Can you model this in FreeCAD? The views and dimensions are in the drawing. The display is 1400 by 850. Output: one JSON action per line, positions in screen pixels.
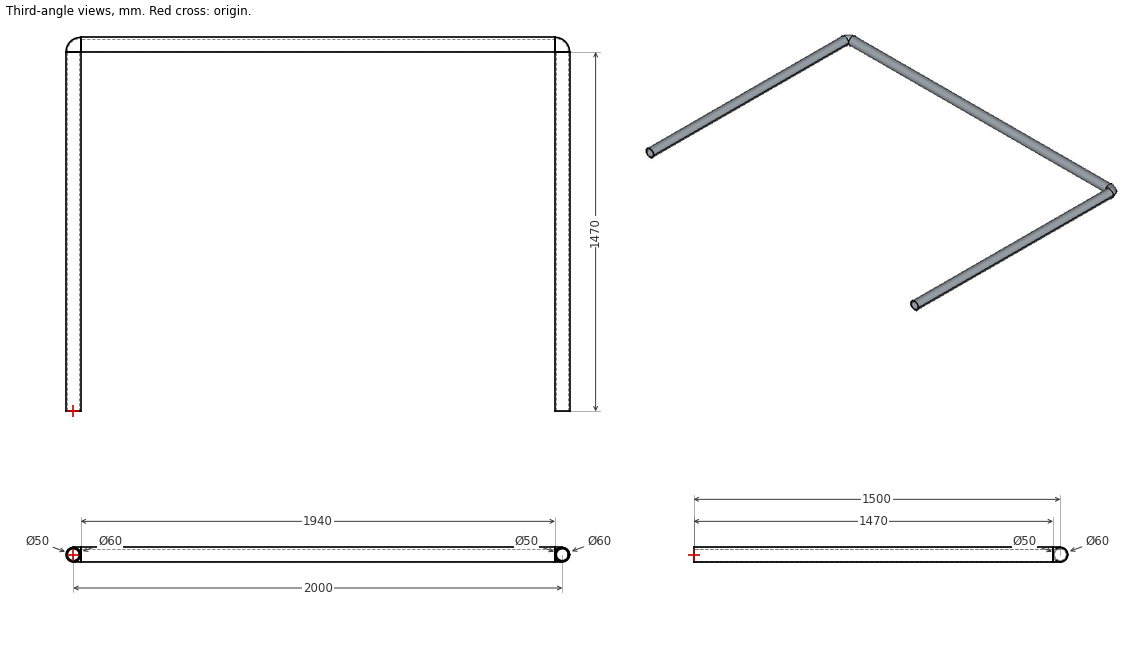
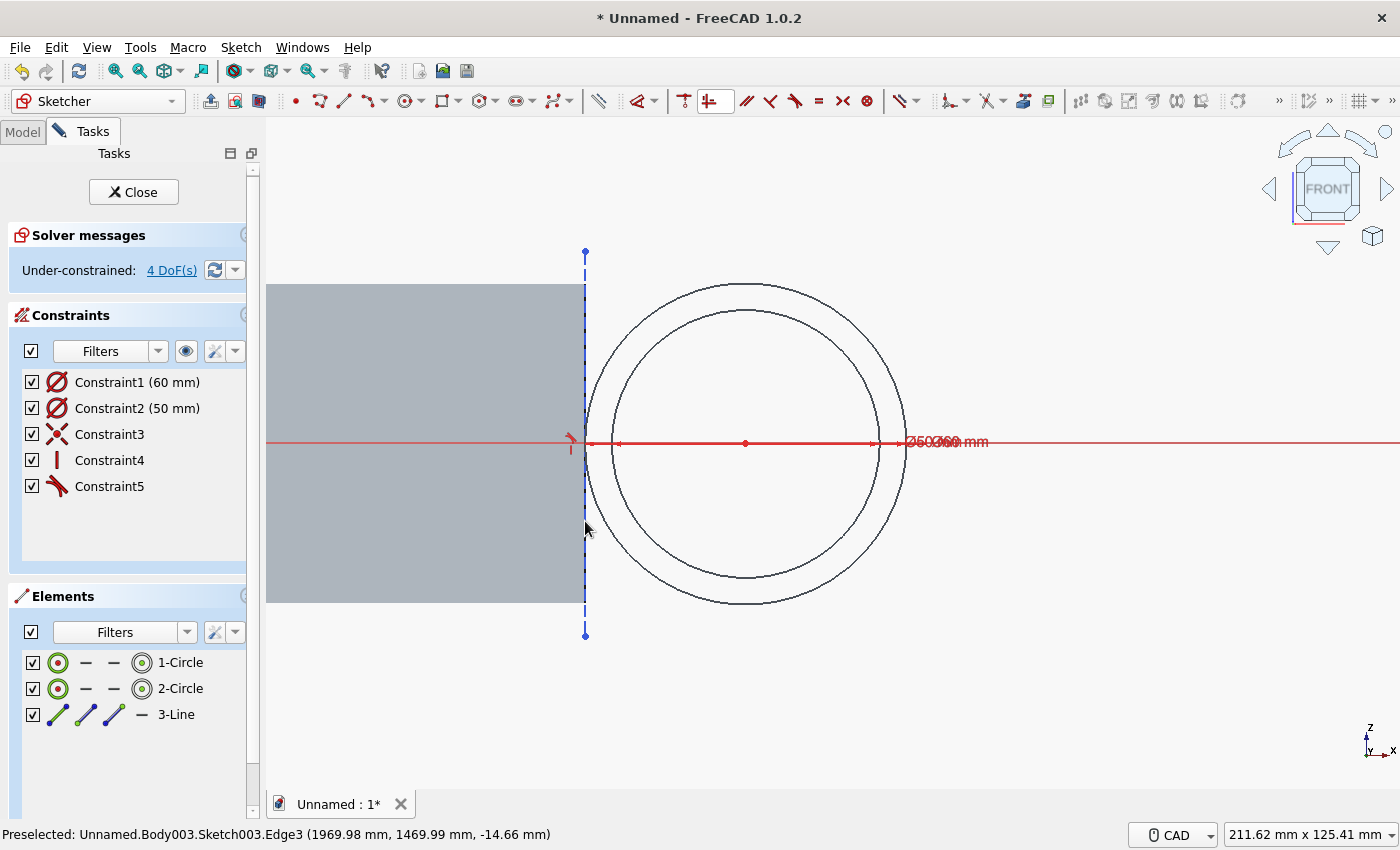
{"action": "left_click", "coordinate": [746, 444]}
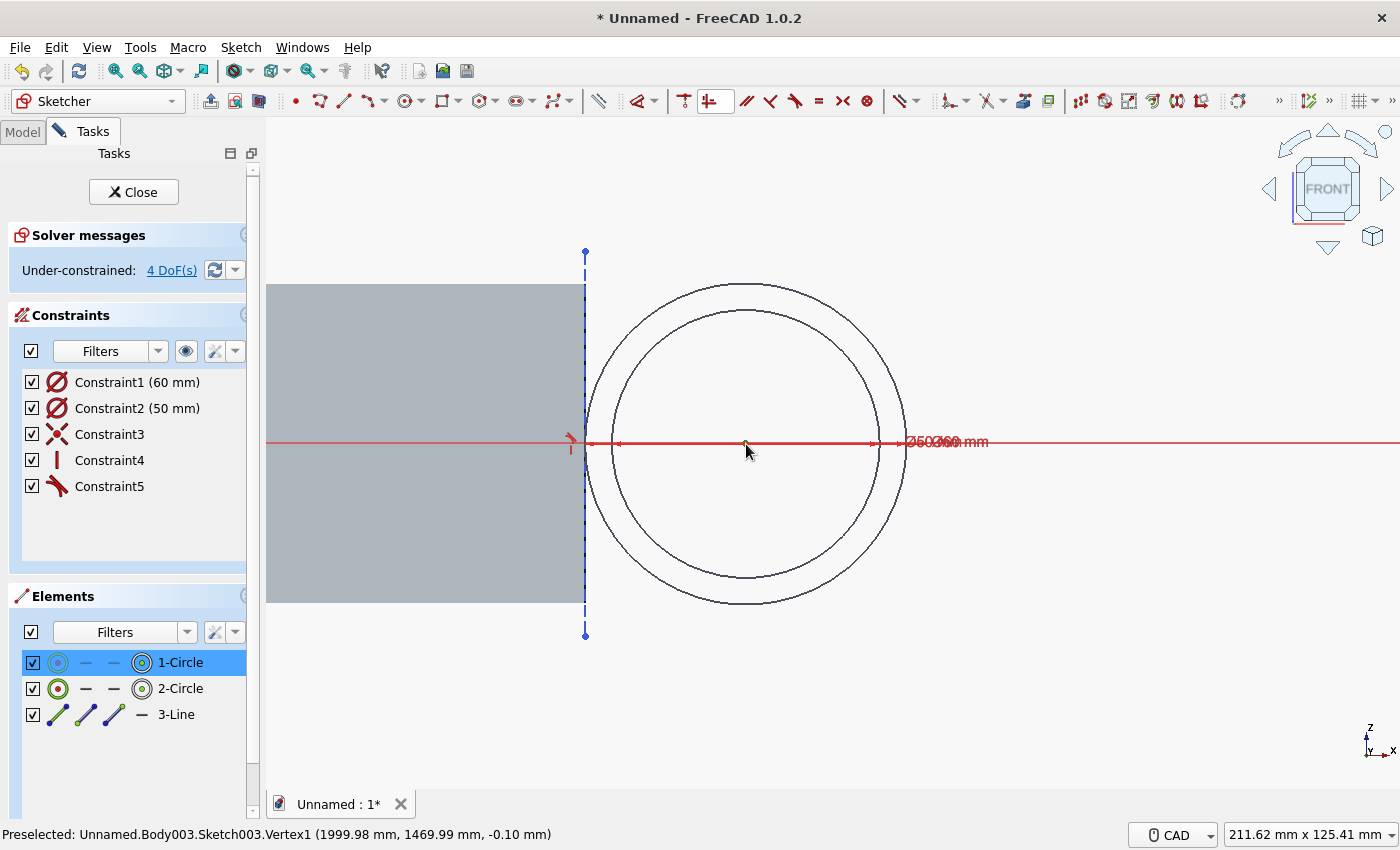
{"action": "left_click", "coordinate": [361, 443]}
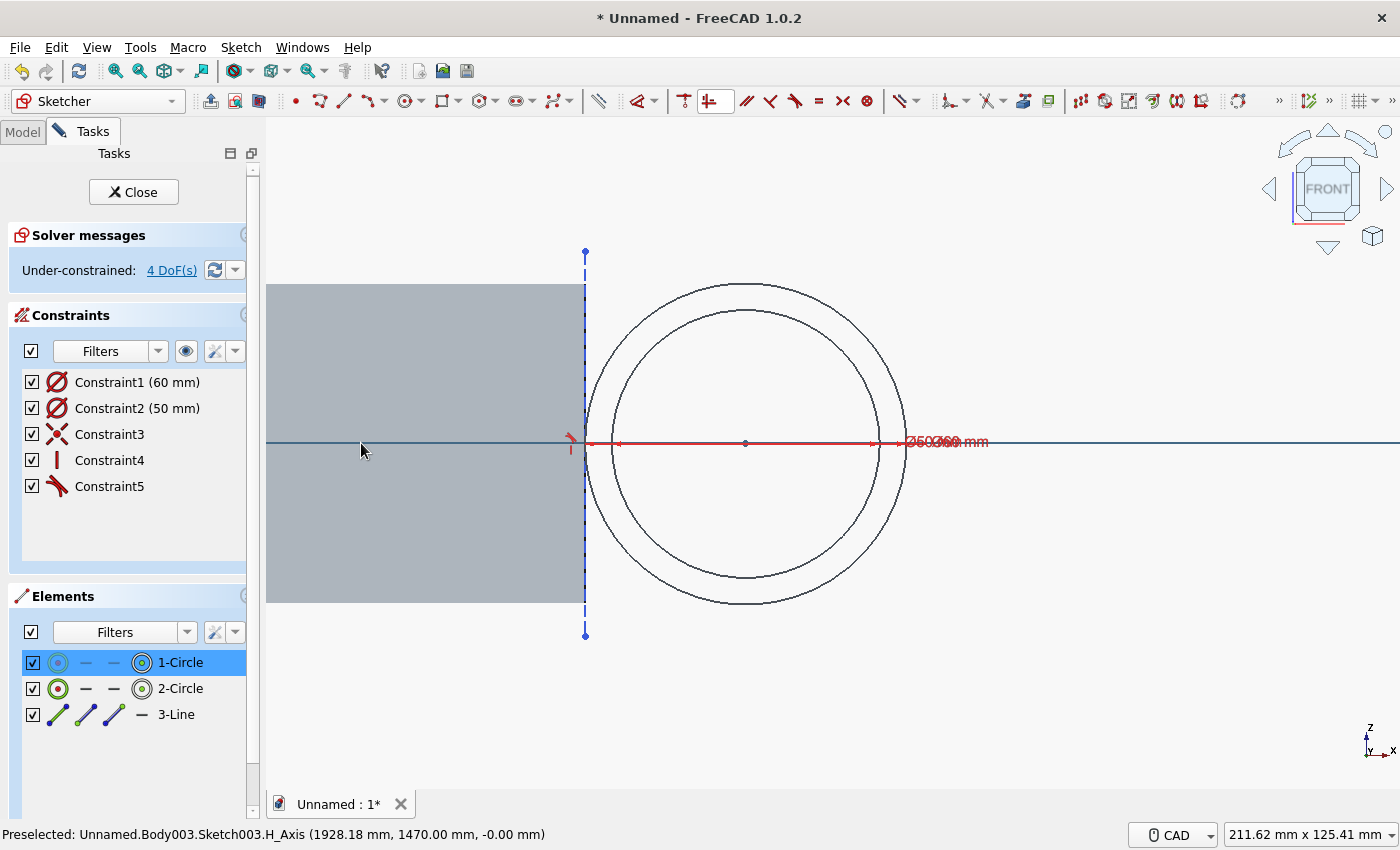
{"action": "key", "text": "c"}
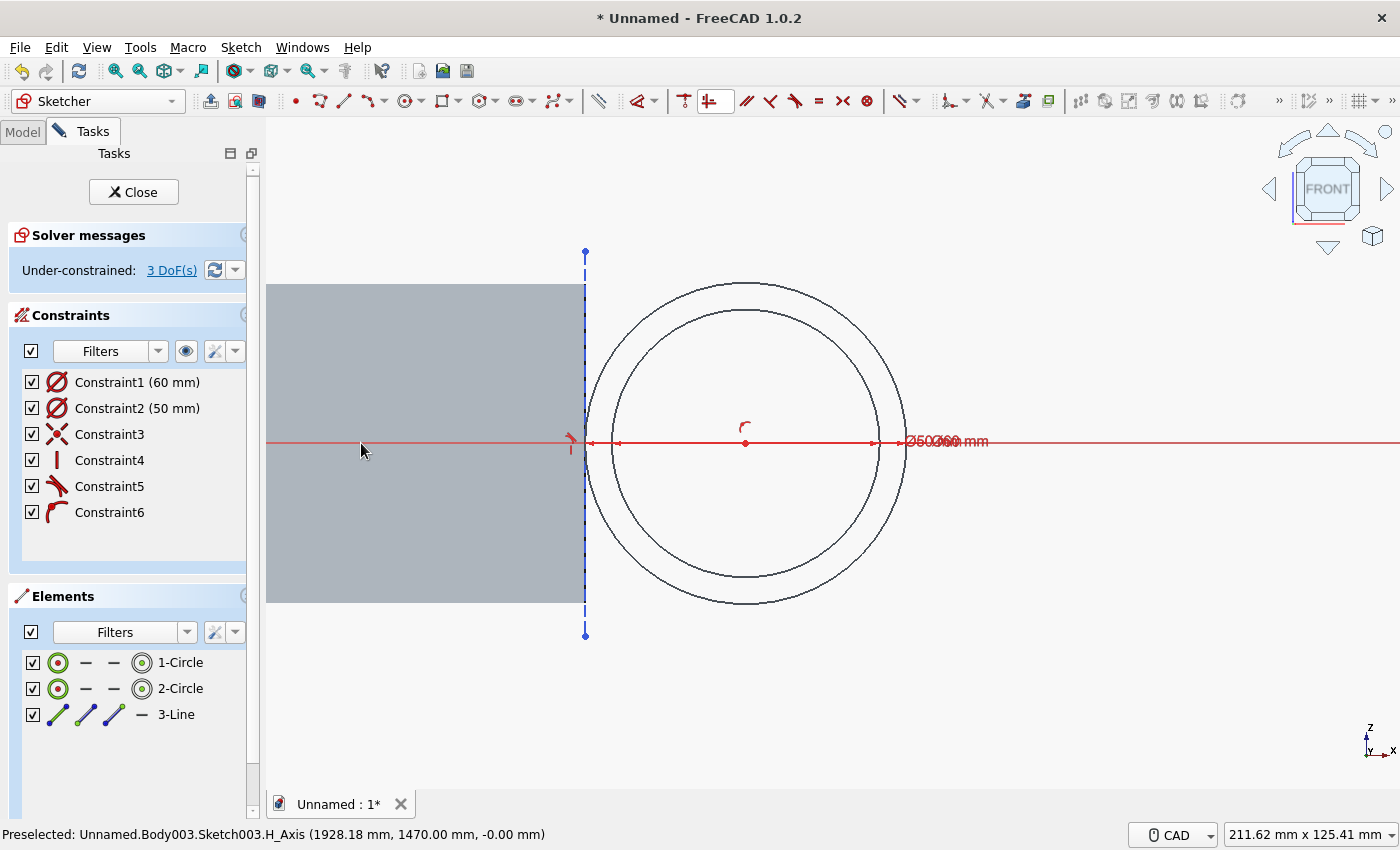
{"action": "left_click", "coordinate": [638, 102]}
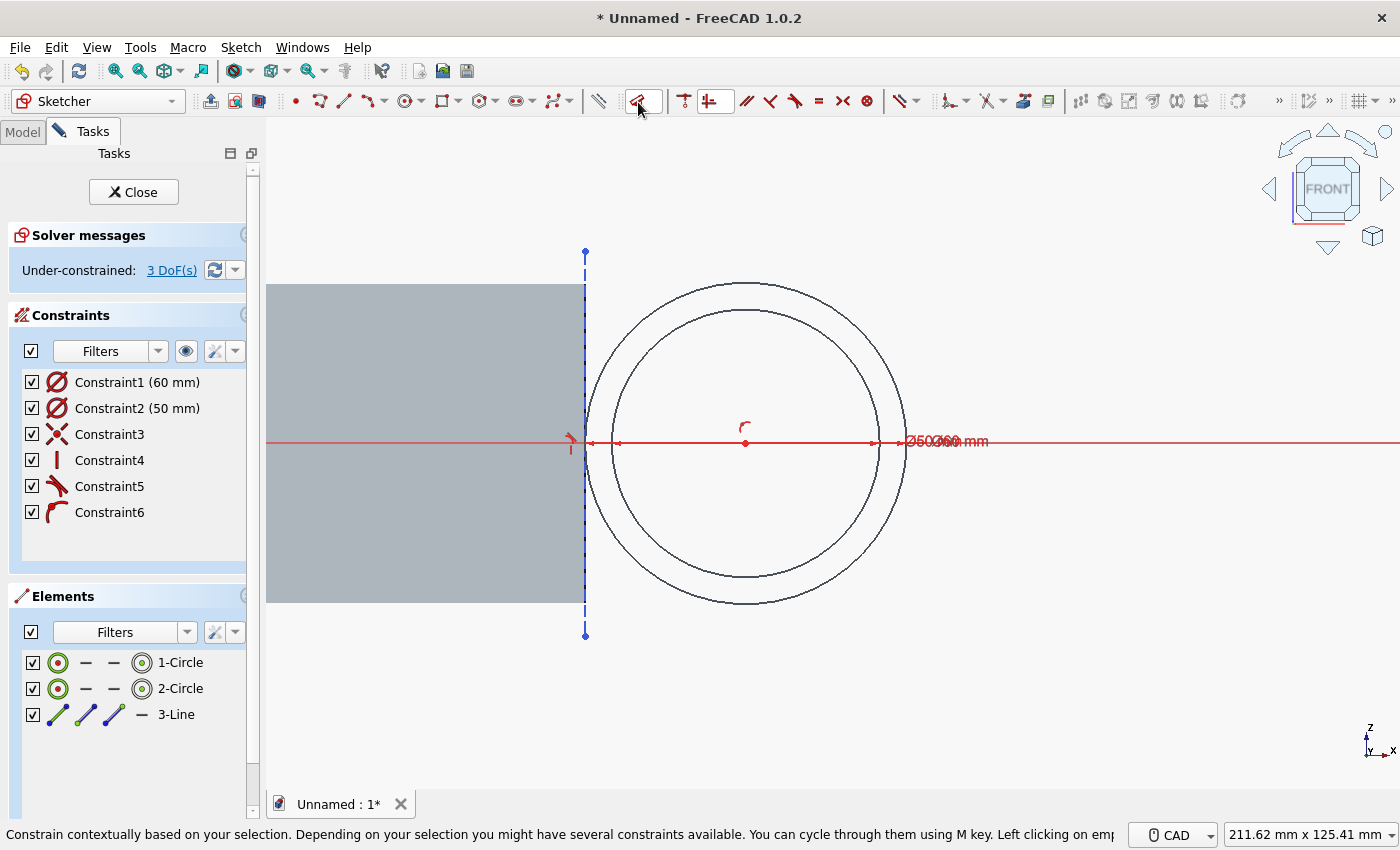
{"action": "left_click", "coordinate": [746, 443]}
{"action": "left_click", "coordinate": [520, 477]}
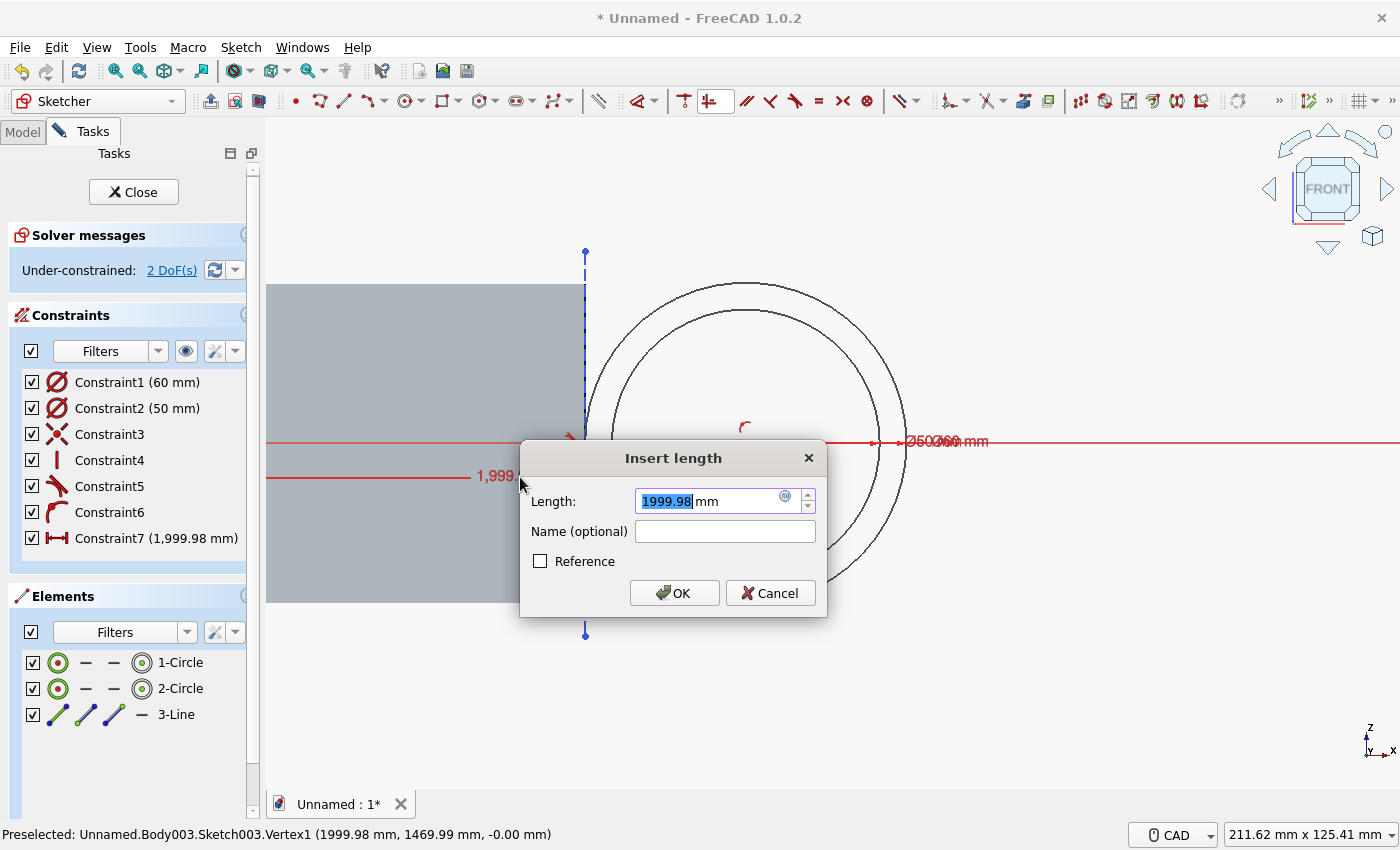
{"action": "type", "text": "2000"}
{"action": "key", "text": "Return"}
{"action": "key", "text": "Escape"}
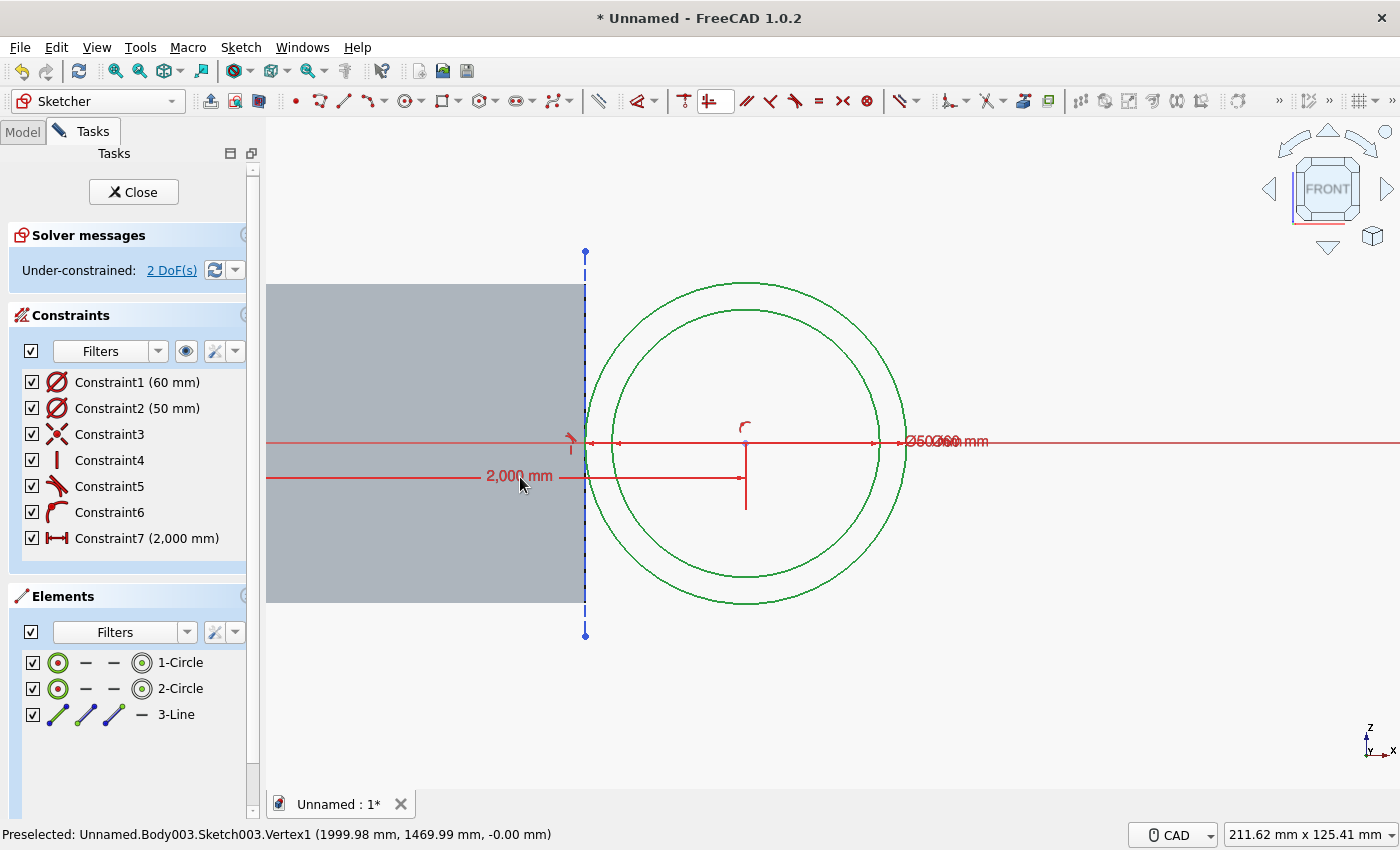
{"action": "left_click", "coordinate": [134, 192]}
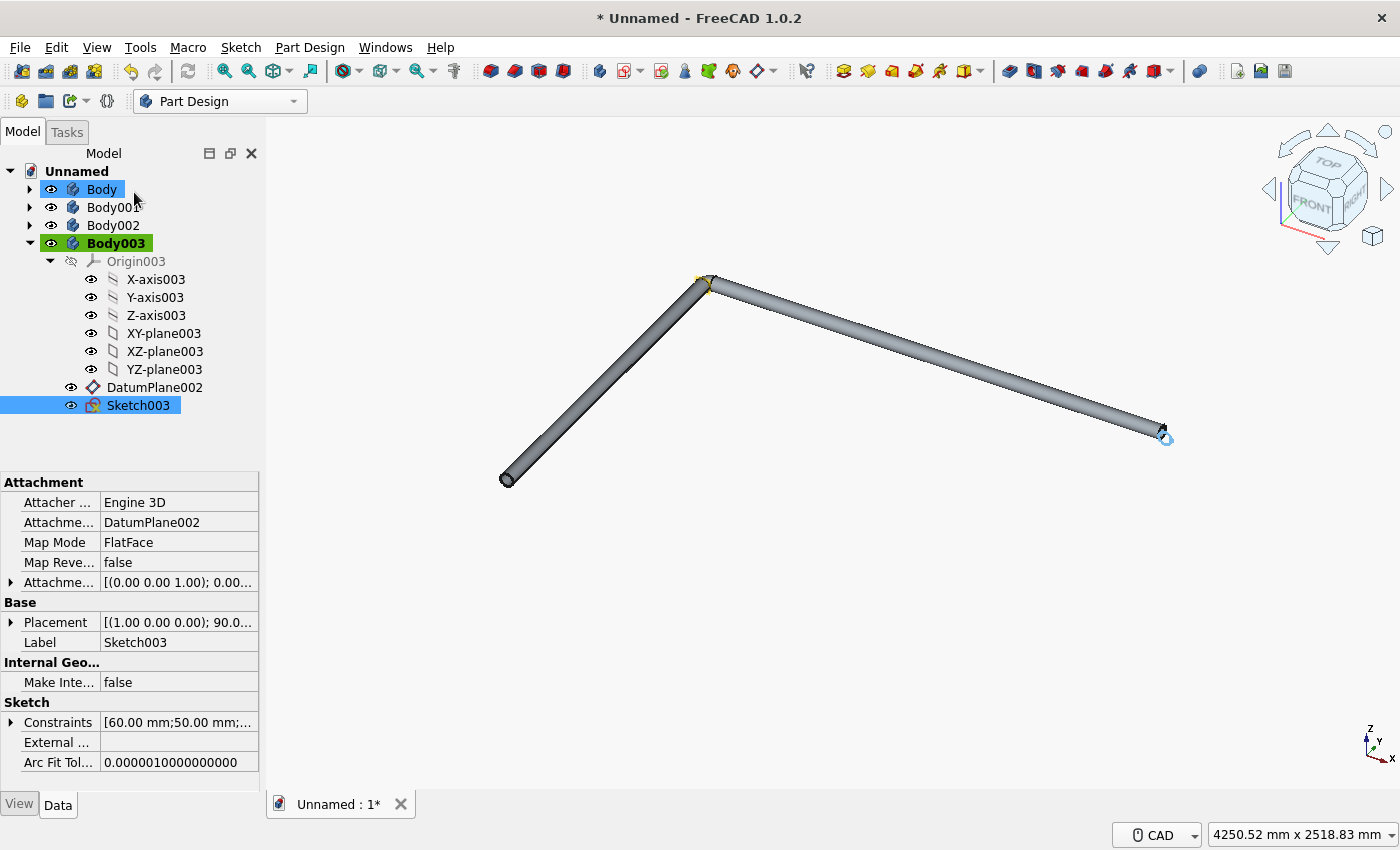
{"action": "left_click", "coordinate": [868, 72]}